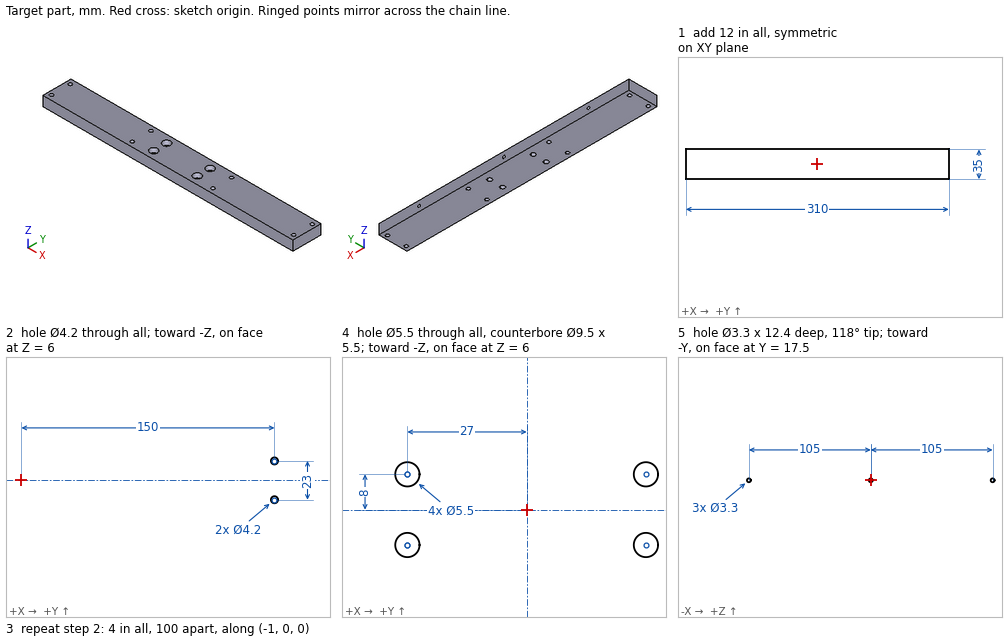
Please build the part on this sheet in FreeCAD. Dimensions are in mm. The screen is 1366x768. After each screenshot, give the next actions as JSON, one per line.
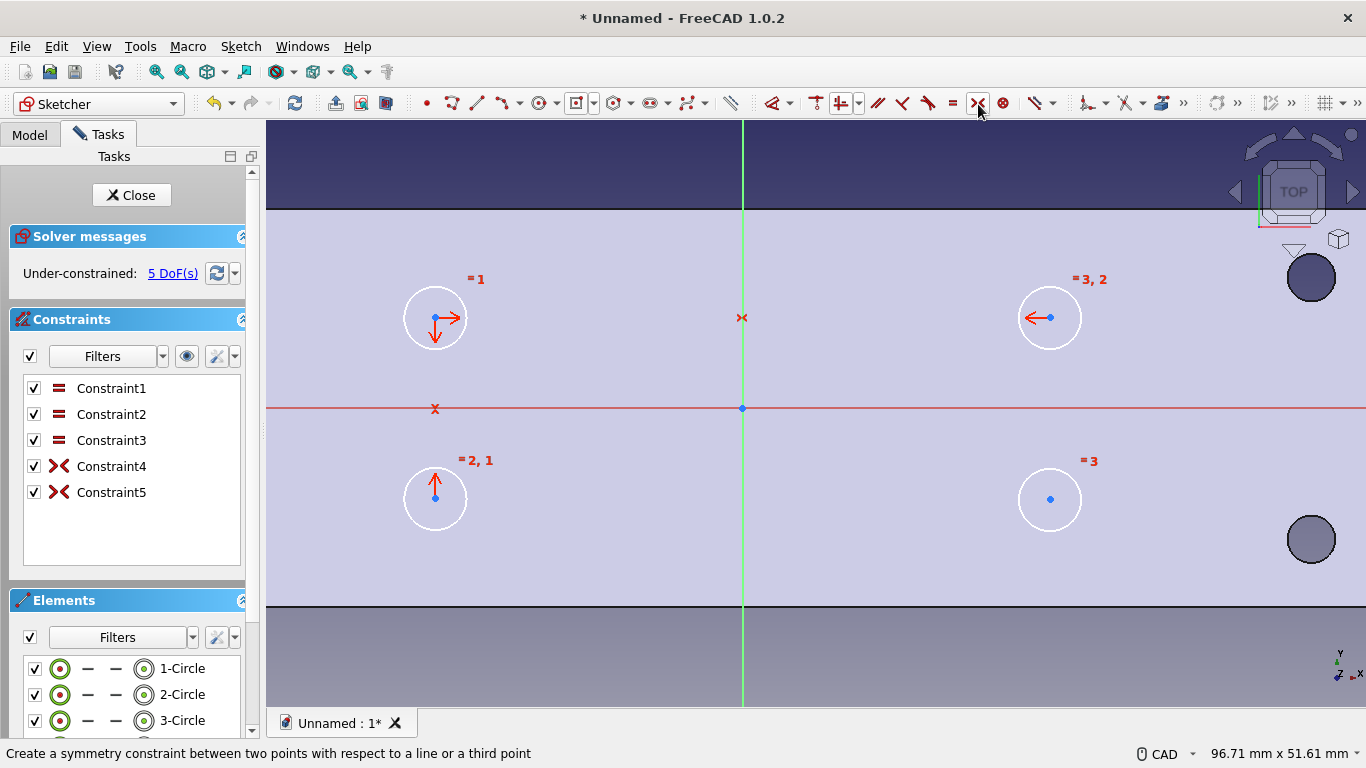
{"action": "left_click", "coordinate": [435, 499]}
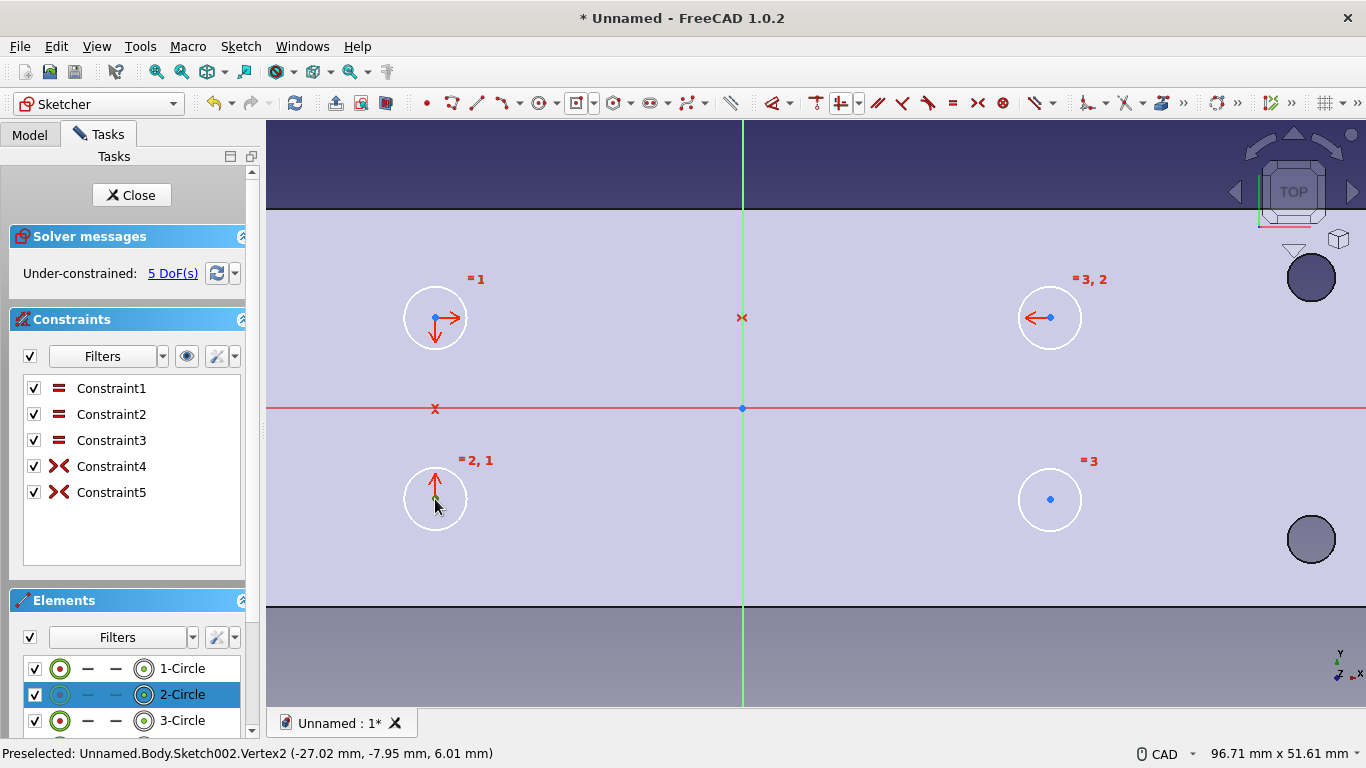
{"action": "left_click", "coordinate": [1050, 500]}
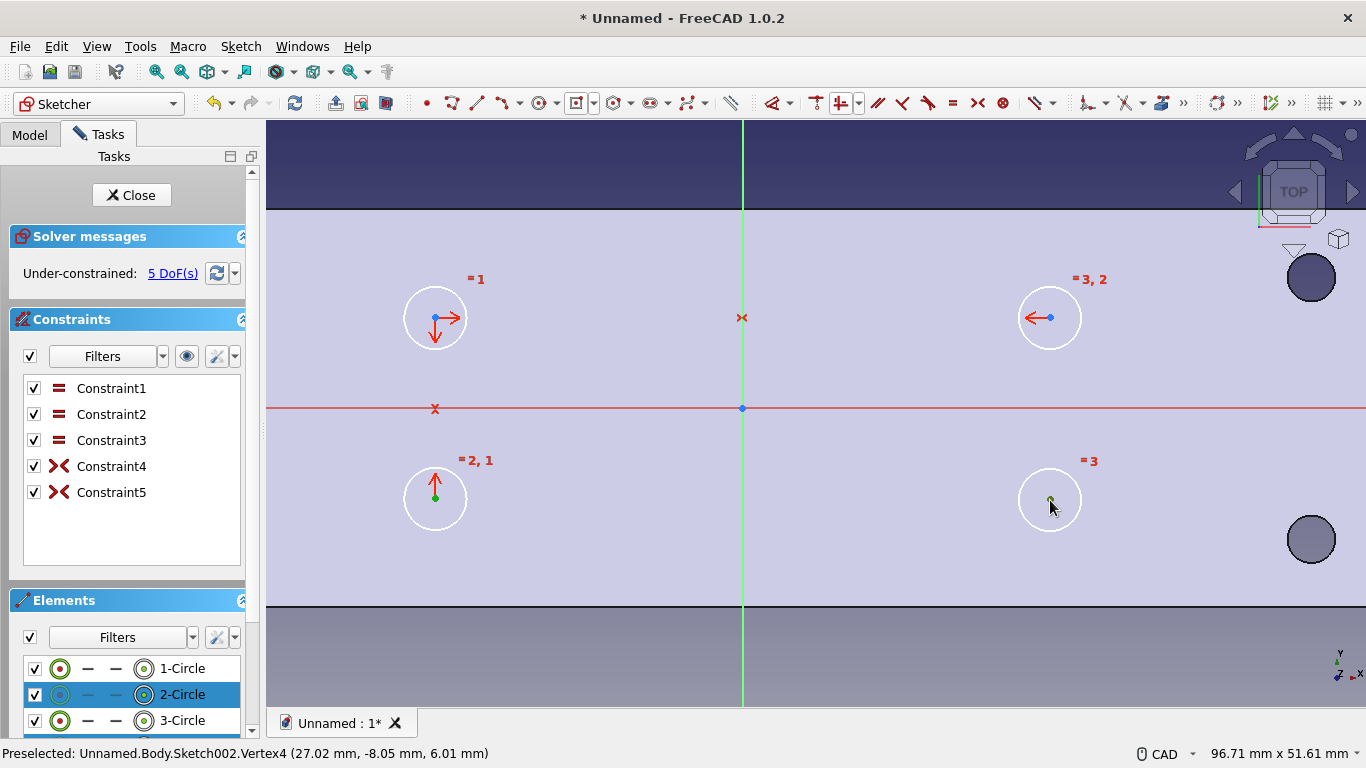
{"action": "left_click", "coordinate": [743, 641]}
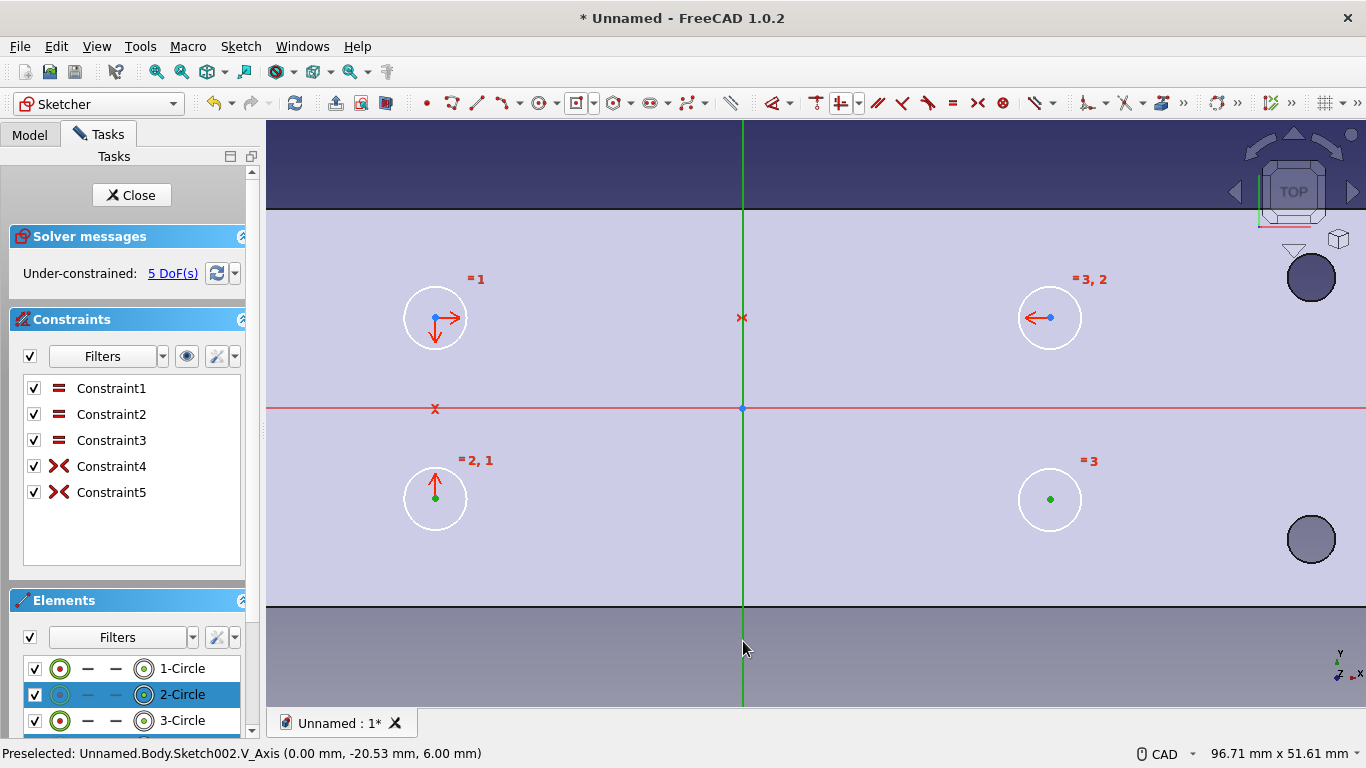
{"action": "left_click", "coordinate": [978, 104]}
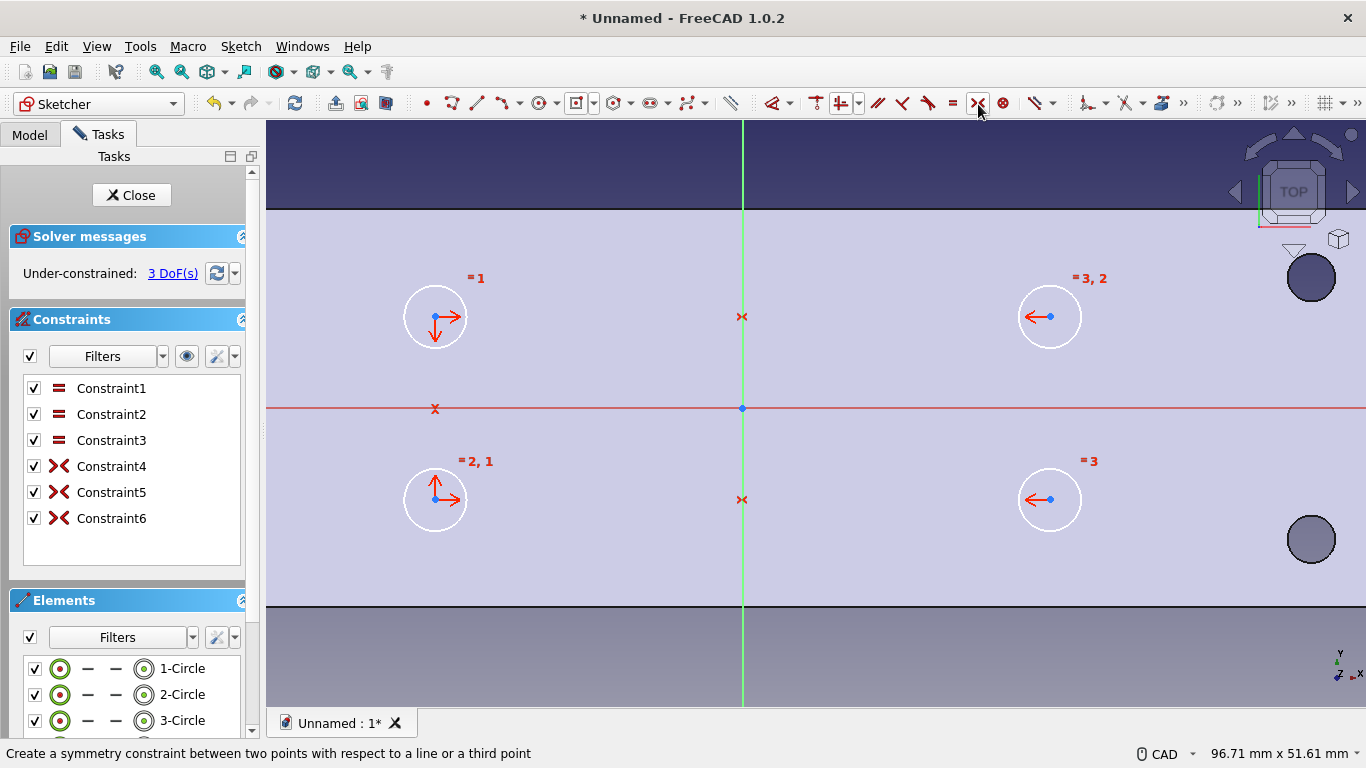
{"action": "left_click", "coordinate": [772, 104]}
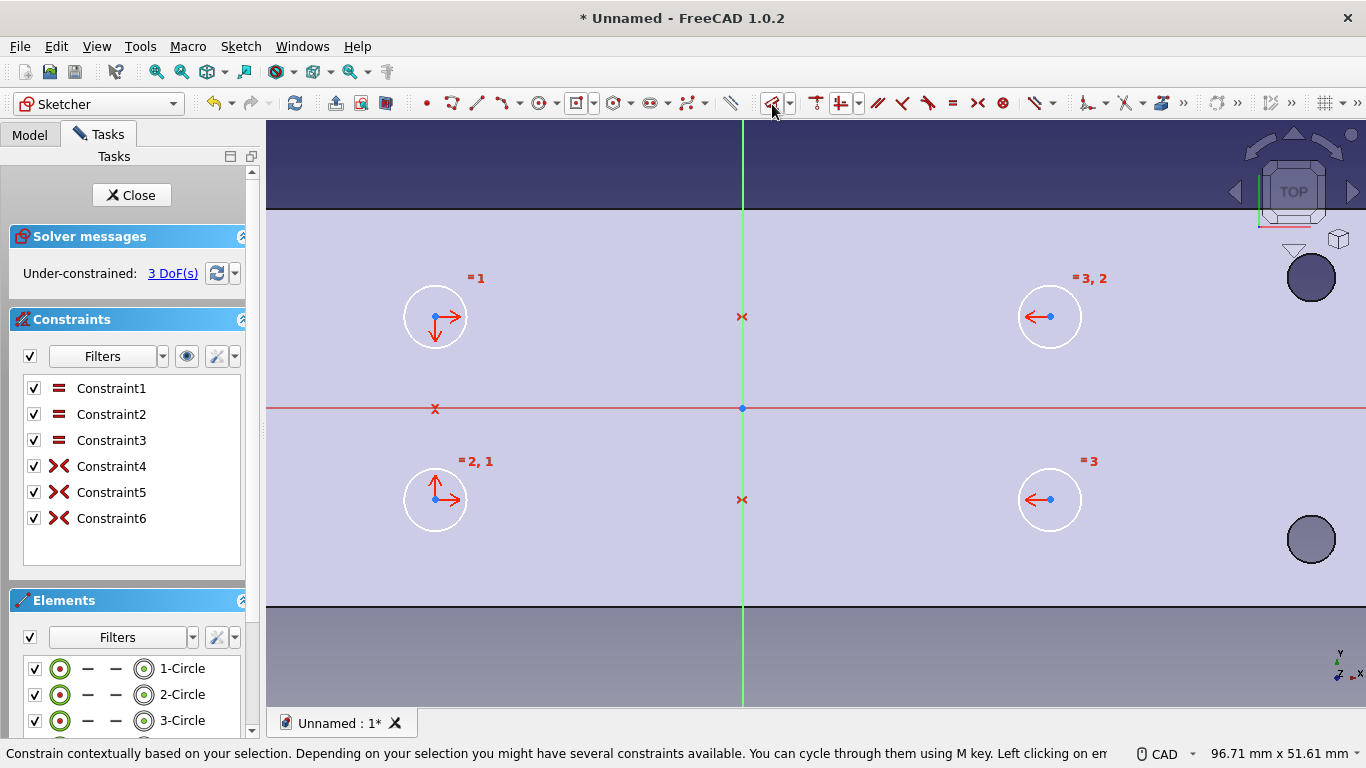
{"action": "left_click", "coordinate": [457, 295]}
{"action": "left_click", "coordinate": [479, 272]}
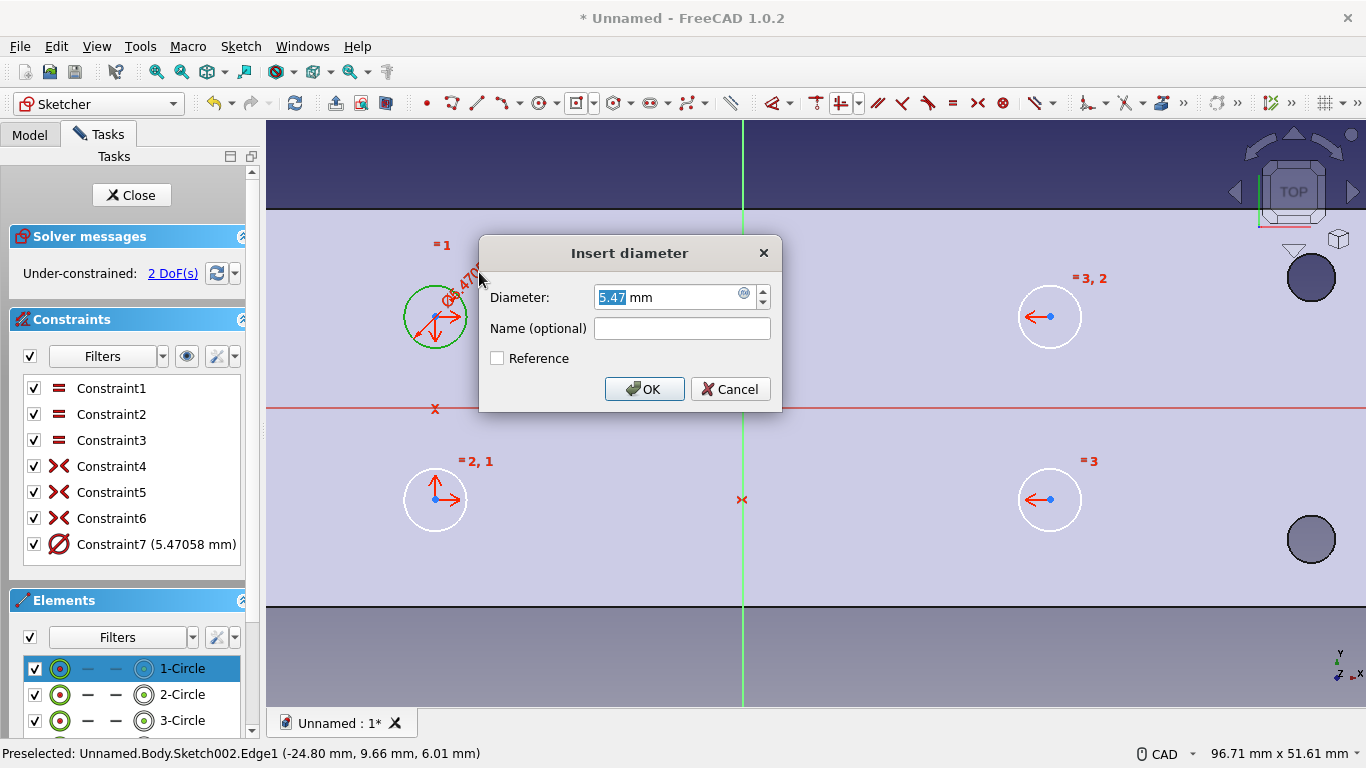
{"action": "type", "text": "5.5"}
{"action": "key", "text": "Return"}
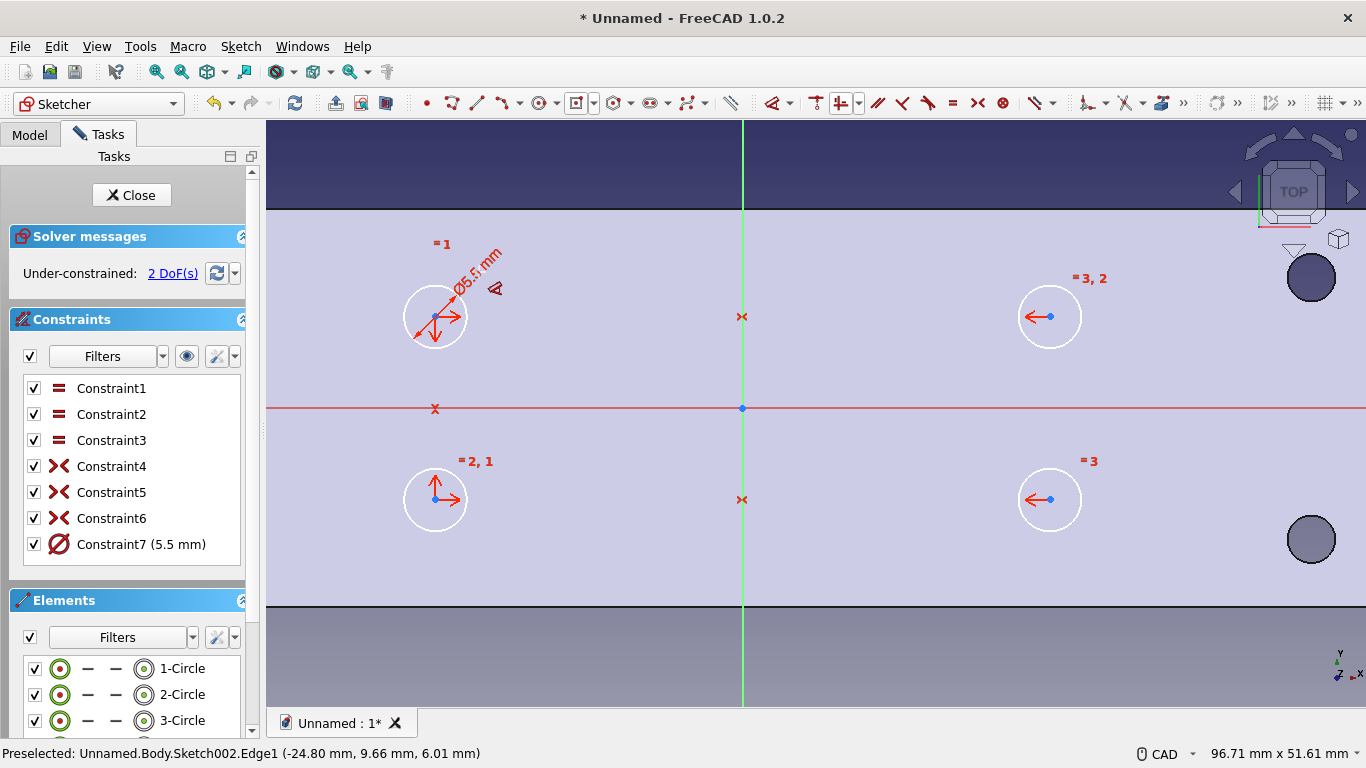
{"action": "left_click", "coordinate": [435, 317]}
{"action": "left_click", "coordinate": [401, 363]}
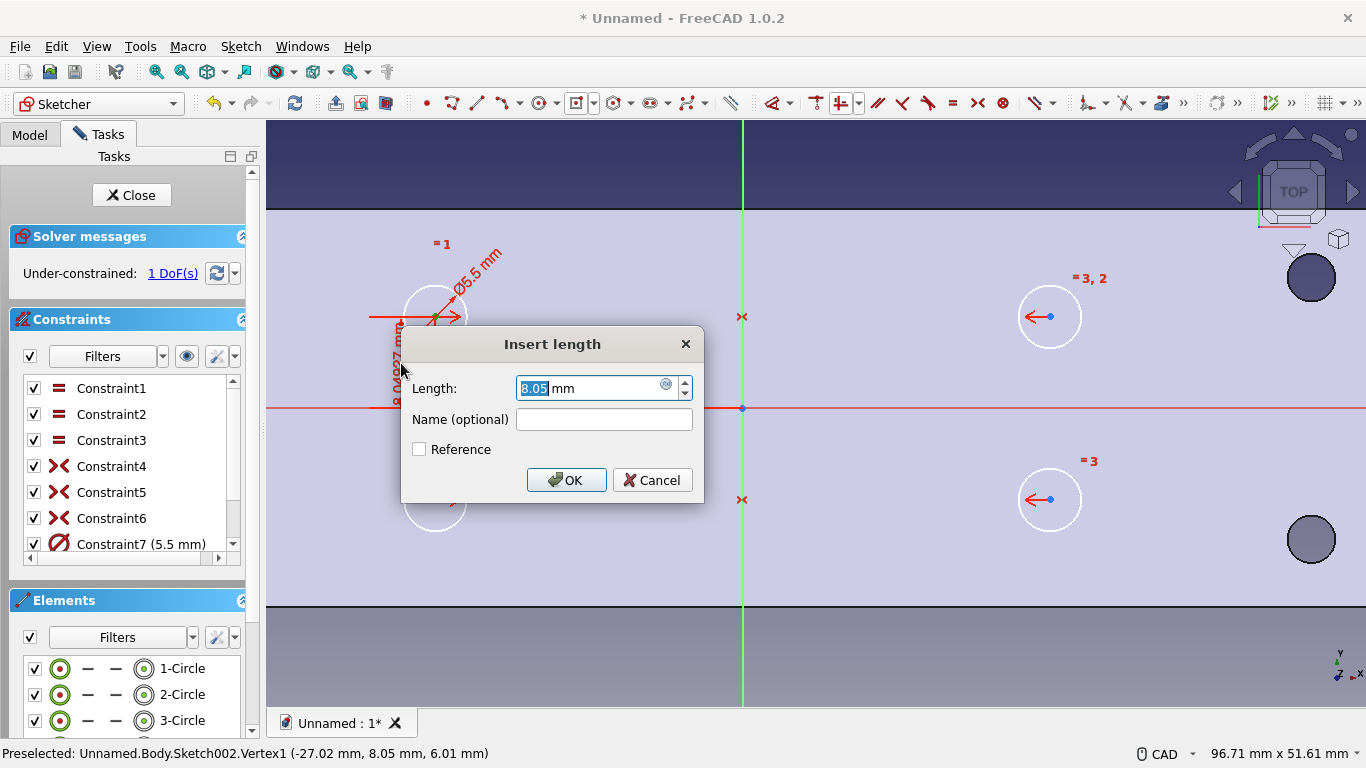
{"action": "type", "text": "8"}
{"action": "key", "text": "Return"}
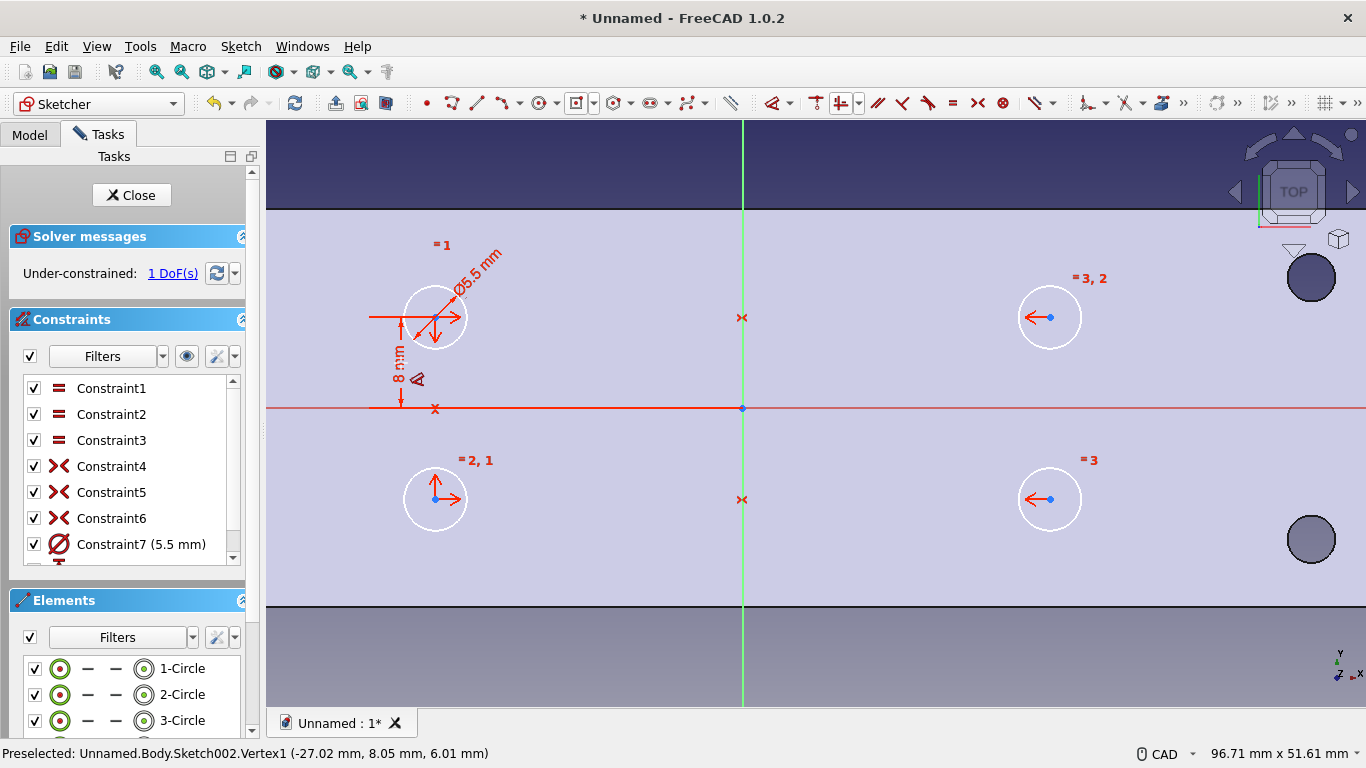
{"action": "left_click", "coordinate": [435, 317]}
{"action": "left_click", "coordinate": [589, 283]}